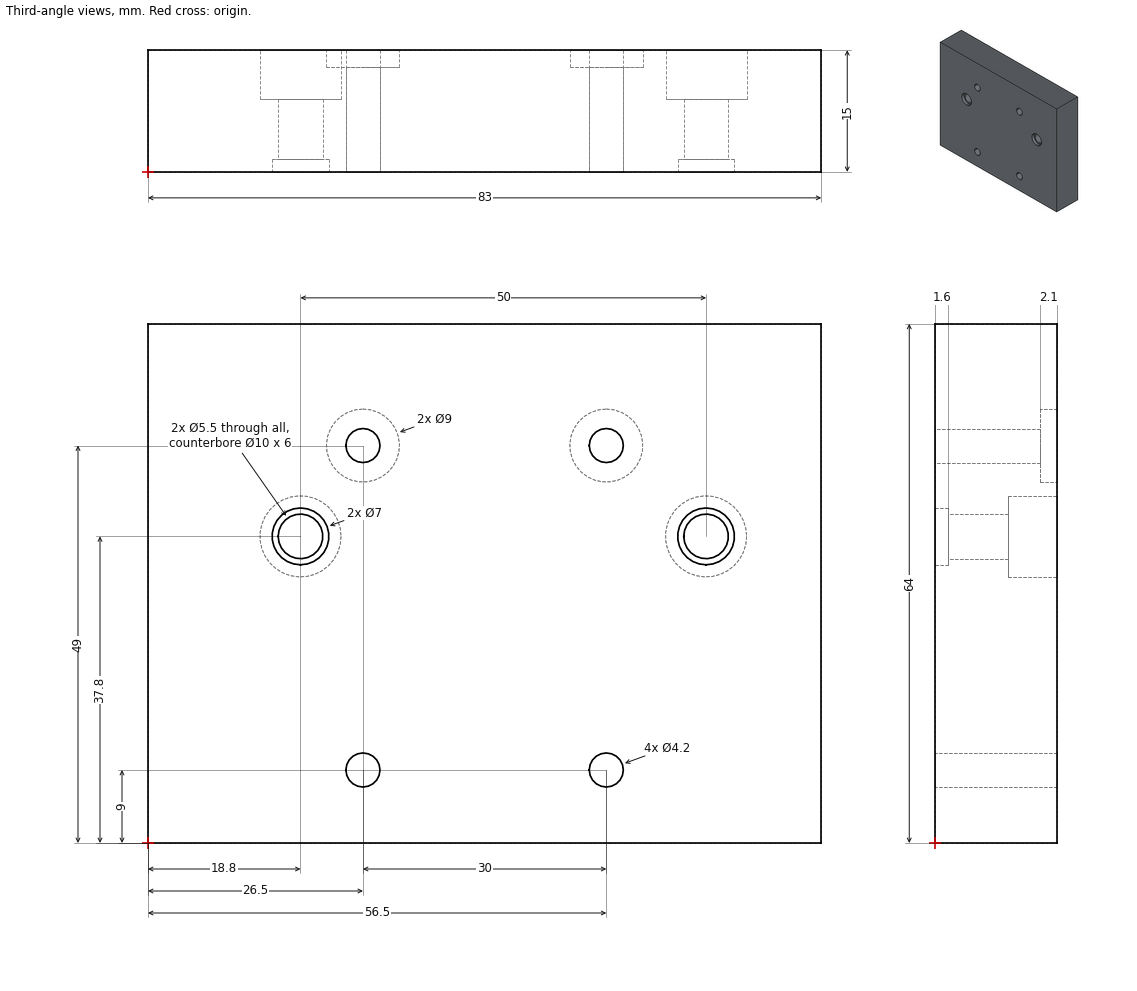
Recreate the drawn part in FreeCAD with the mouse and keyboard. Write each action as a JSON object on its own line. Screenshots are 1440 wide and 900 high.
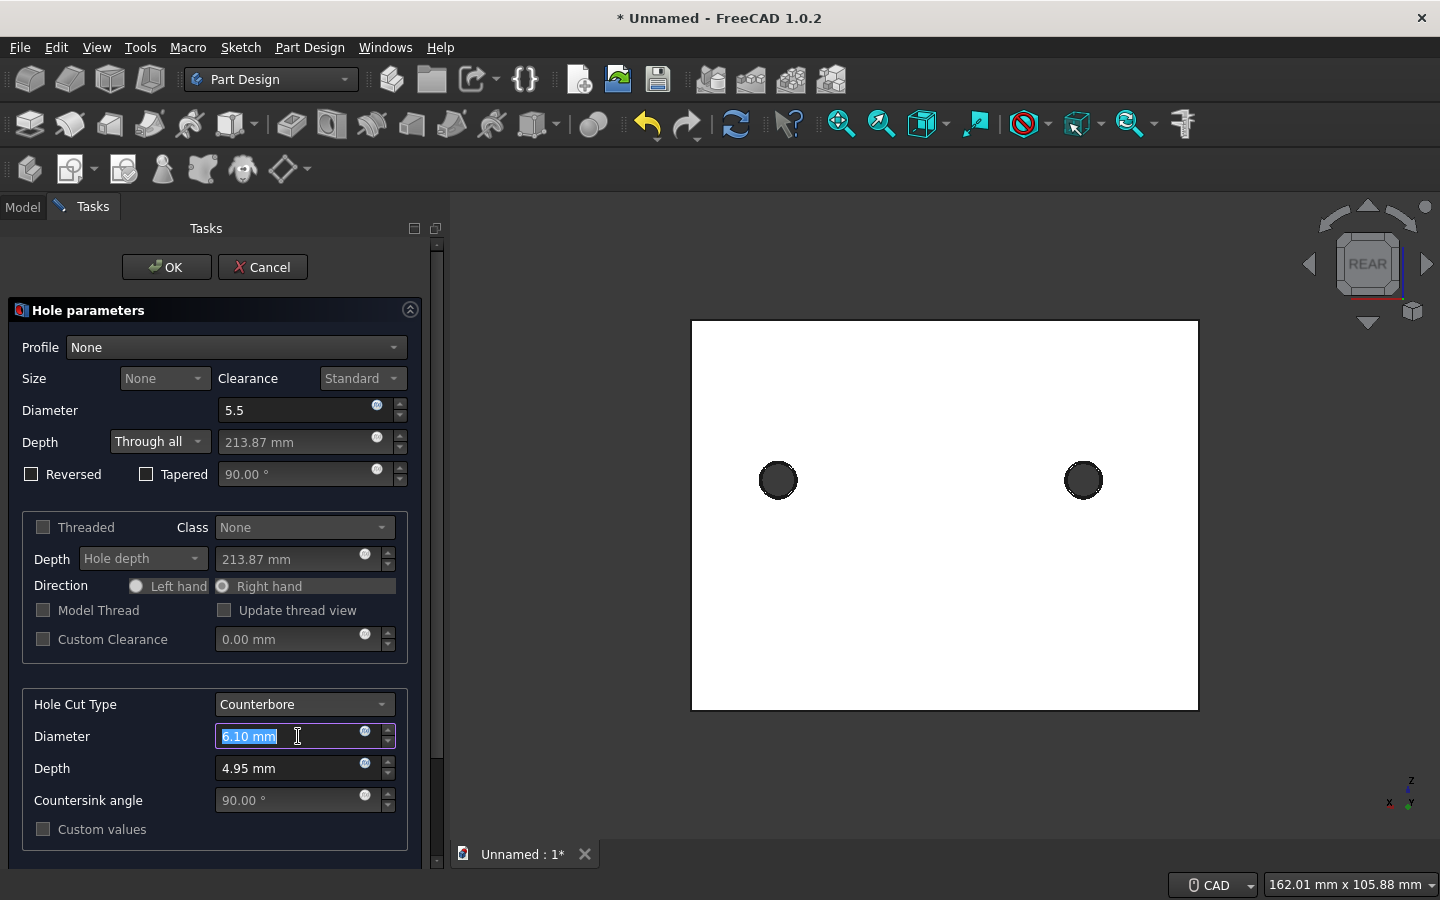
{"action": "type", "text": "10"}
{"action": "key", "text": "Tab"}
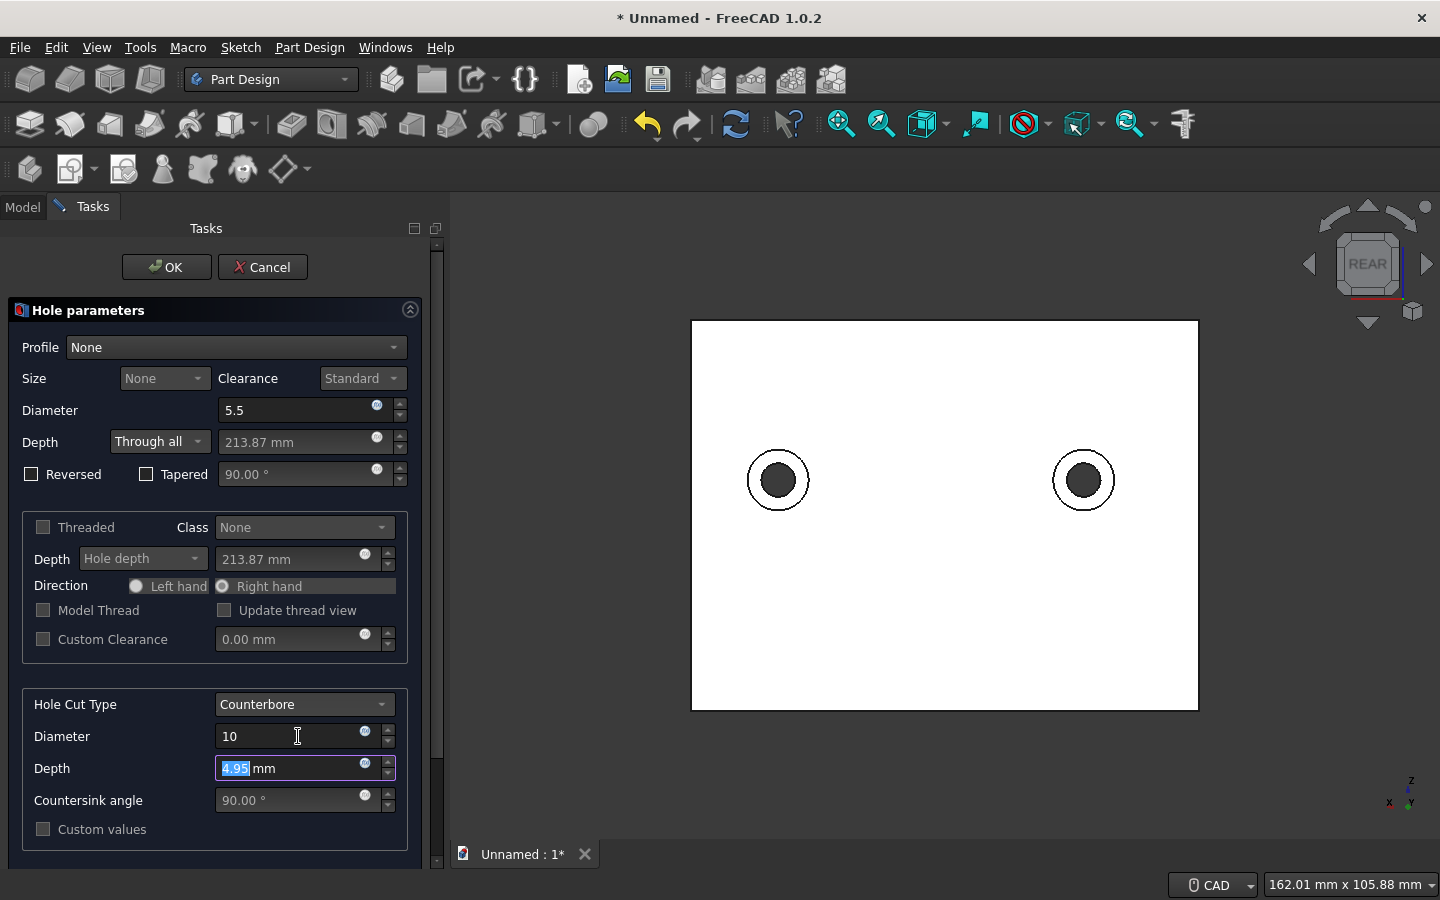
{"action": "type", "text": "6"}
{"action": "key", "text": "Tab"}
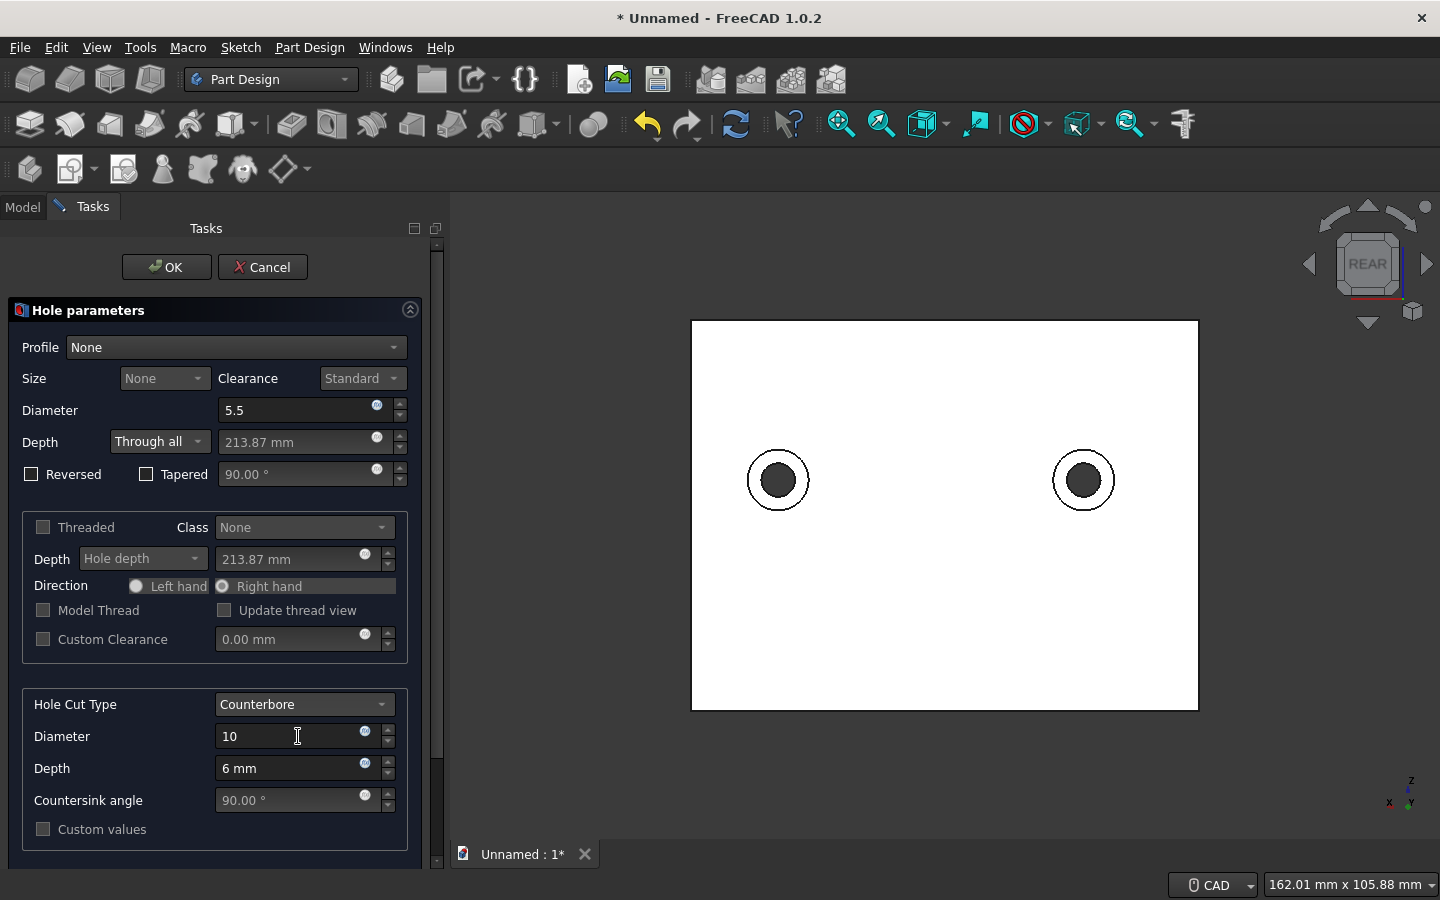
{"action": "left_click", "coordinate": [167, 267]}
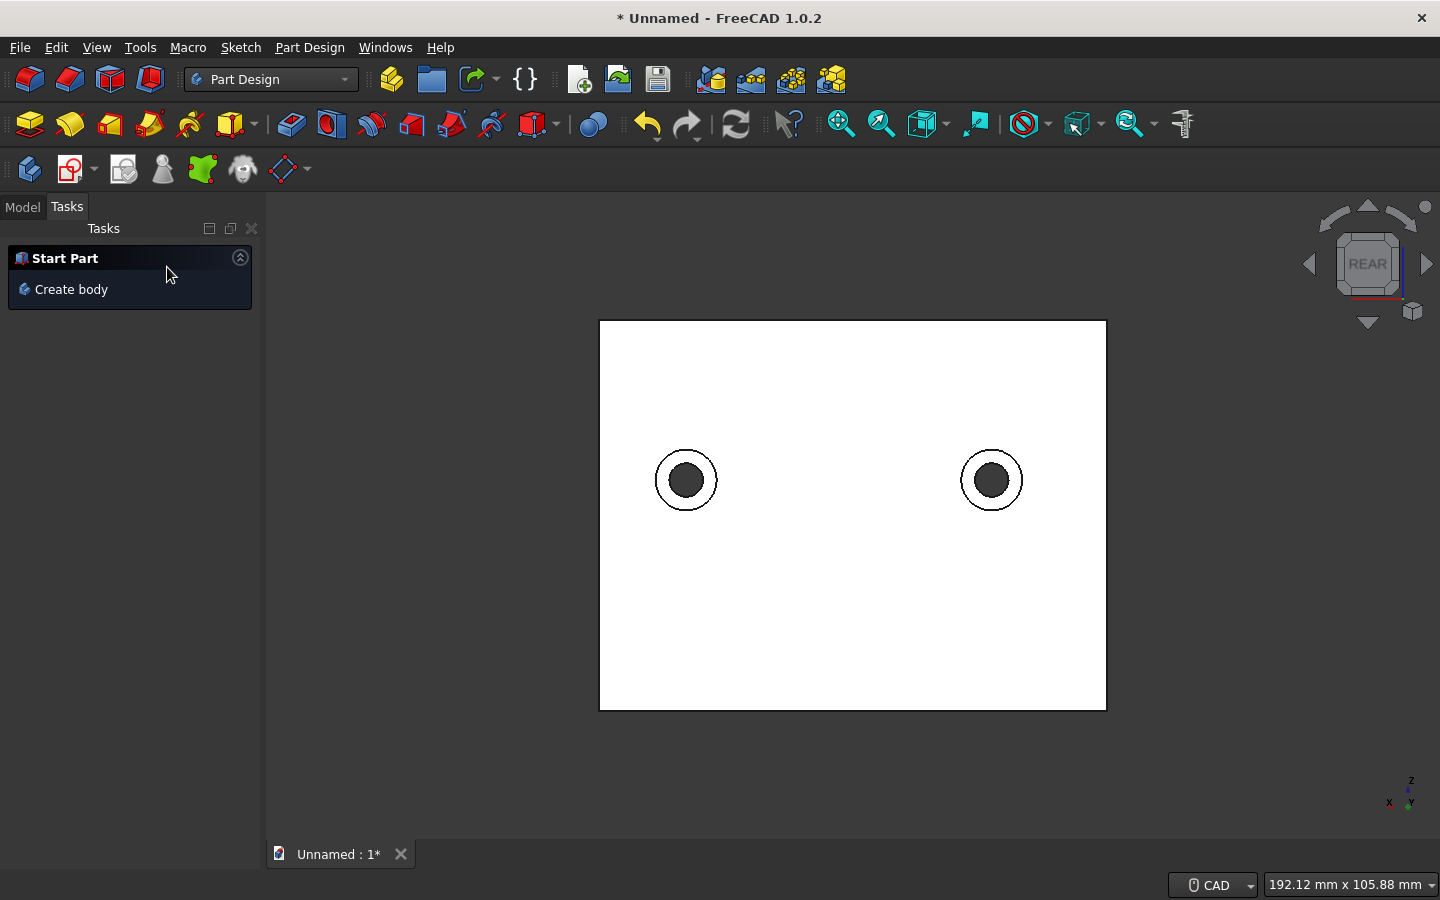
{"action": "left_click", "coordinate": [70, 170]}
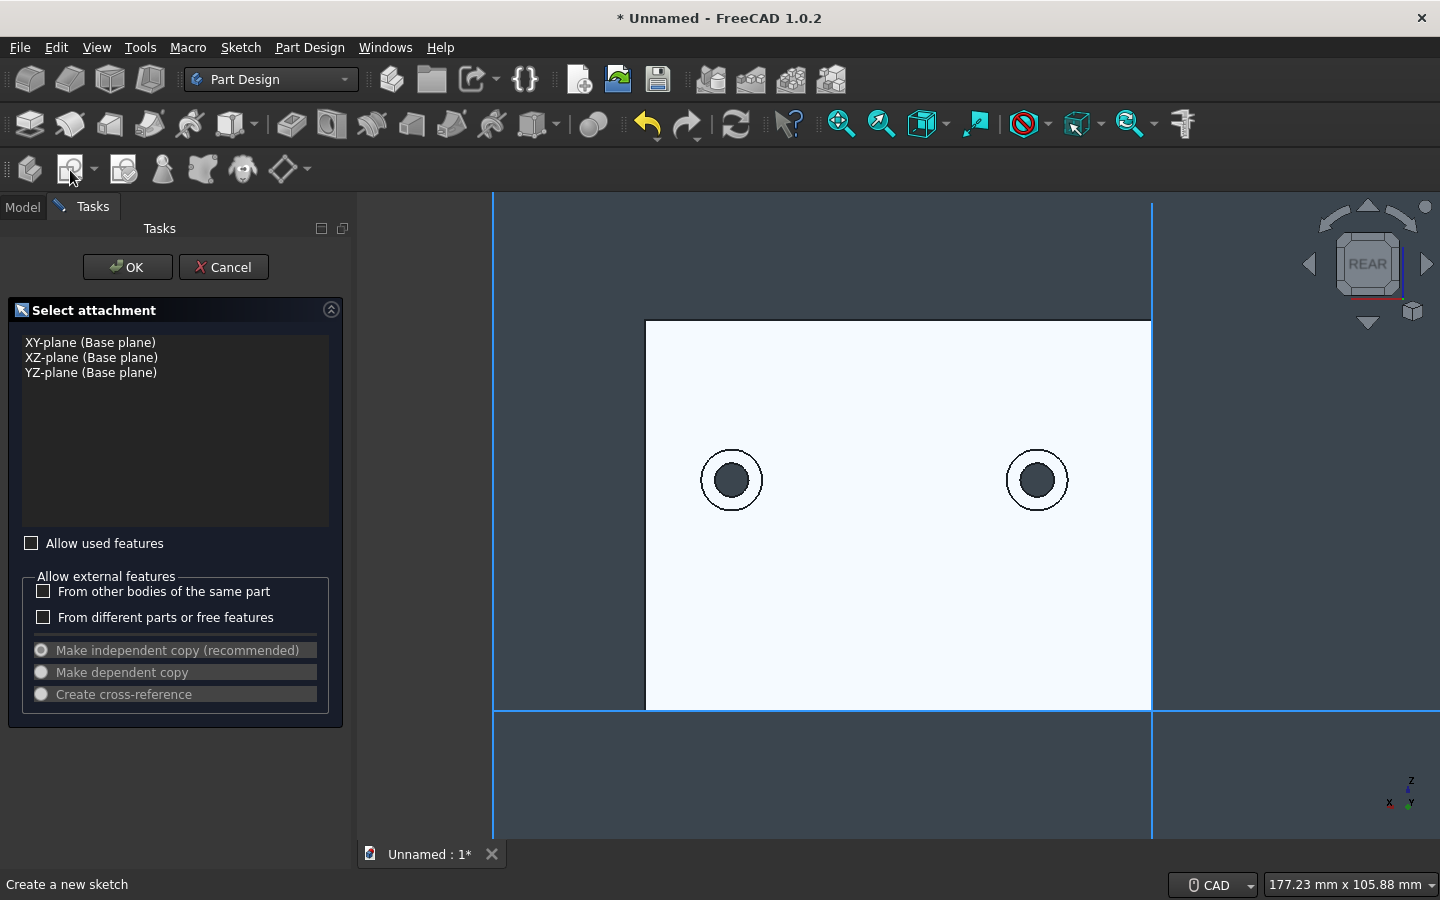
{"action": "left_click", "coordinate": [82, 358]}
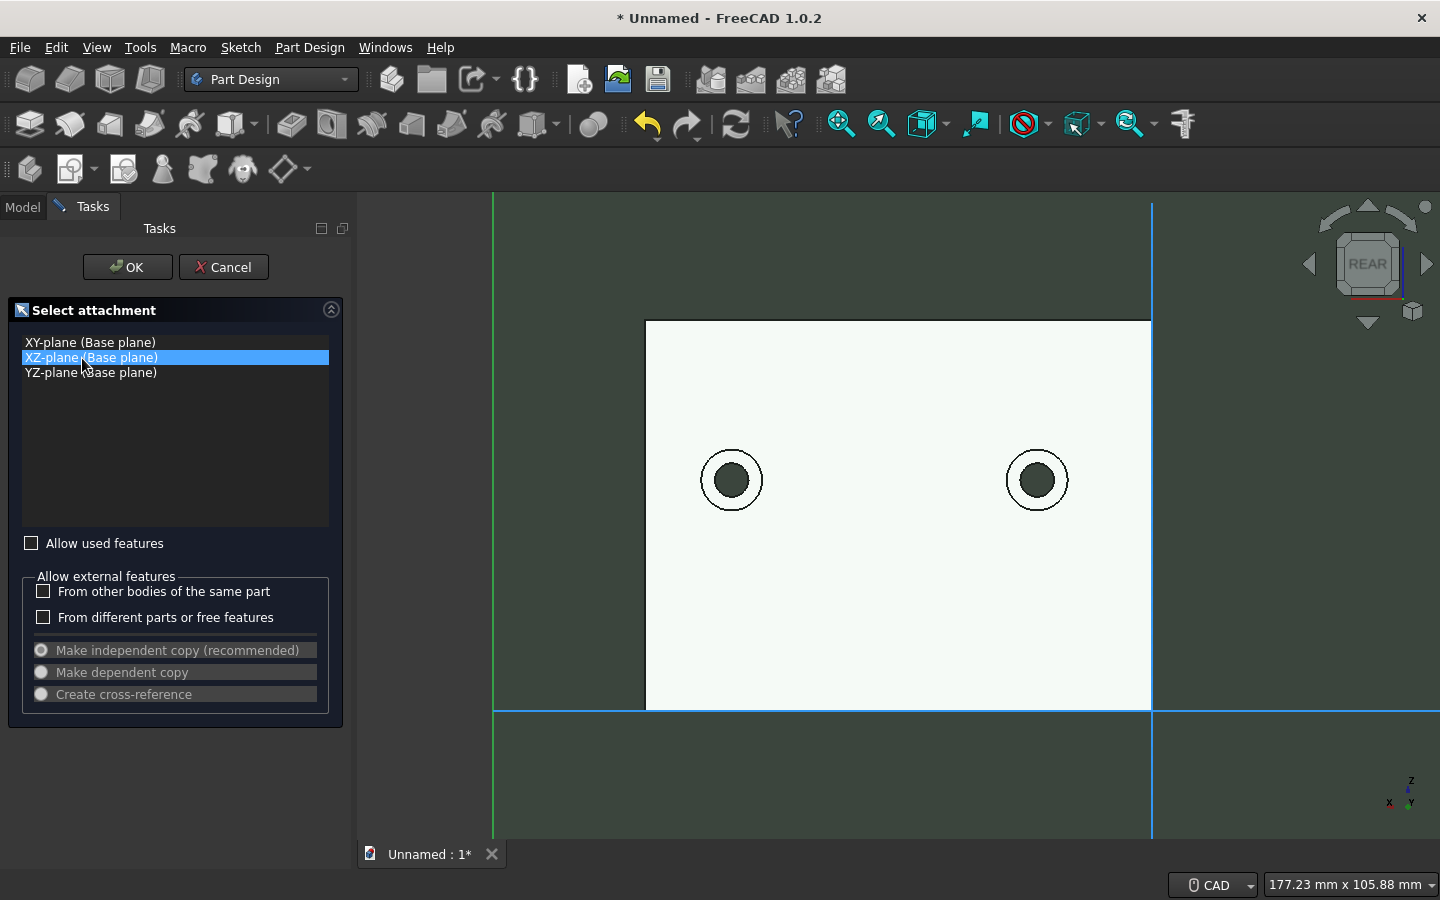
{"action": "left_click", "coordinate": [128, 267]}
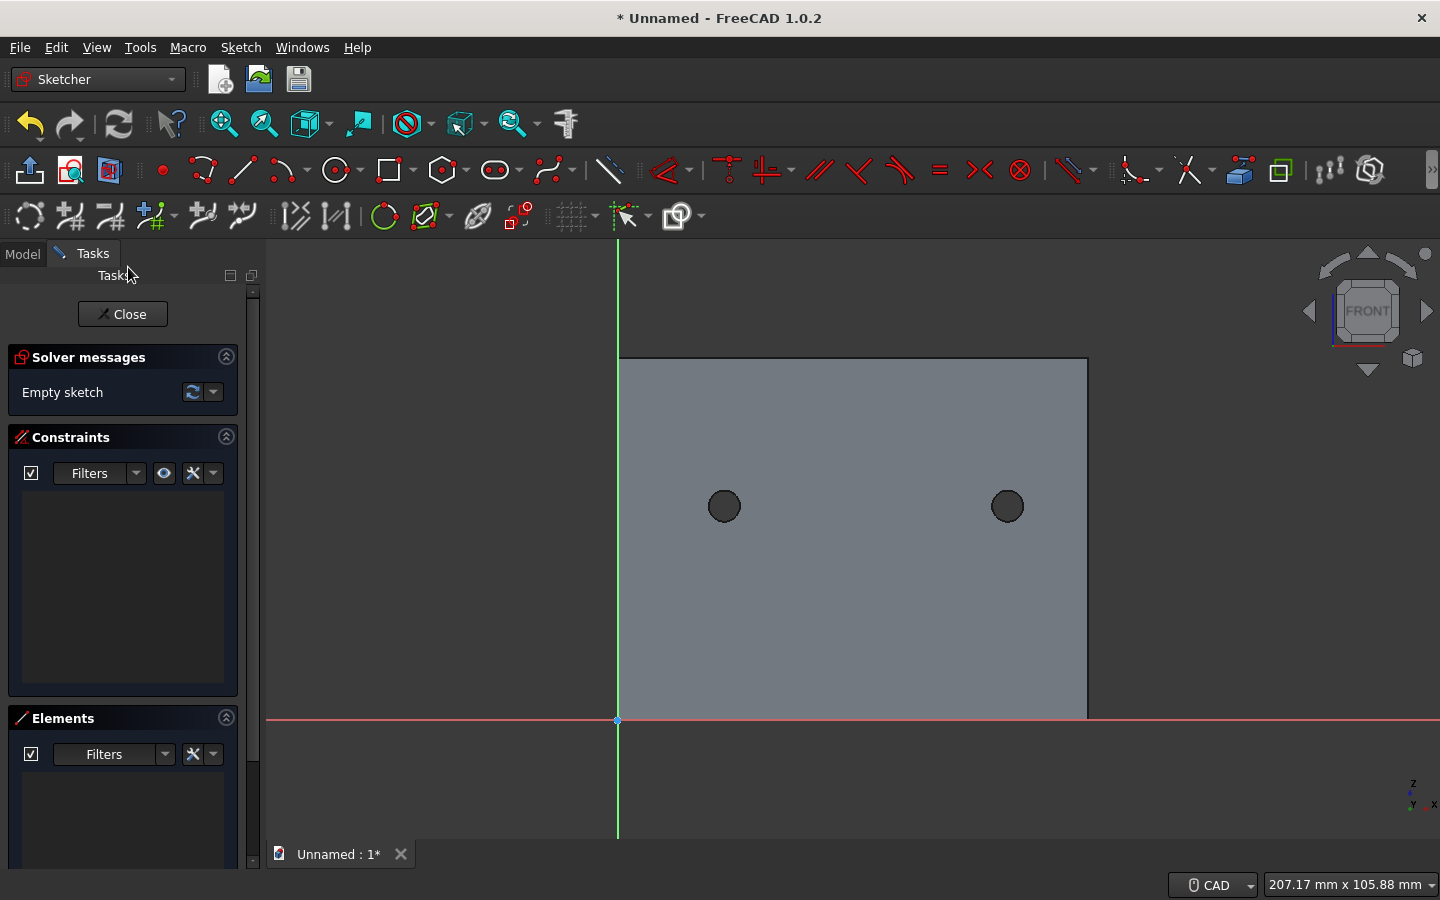
{"action": "scroll", "coordinate": [900, 734], "scroll_direction": "up", "scroll_amount": 2}